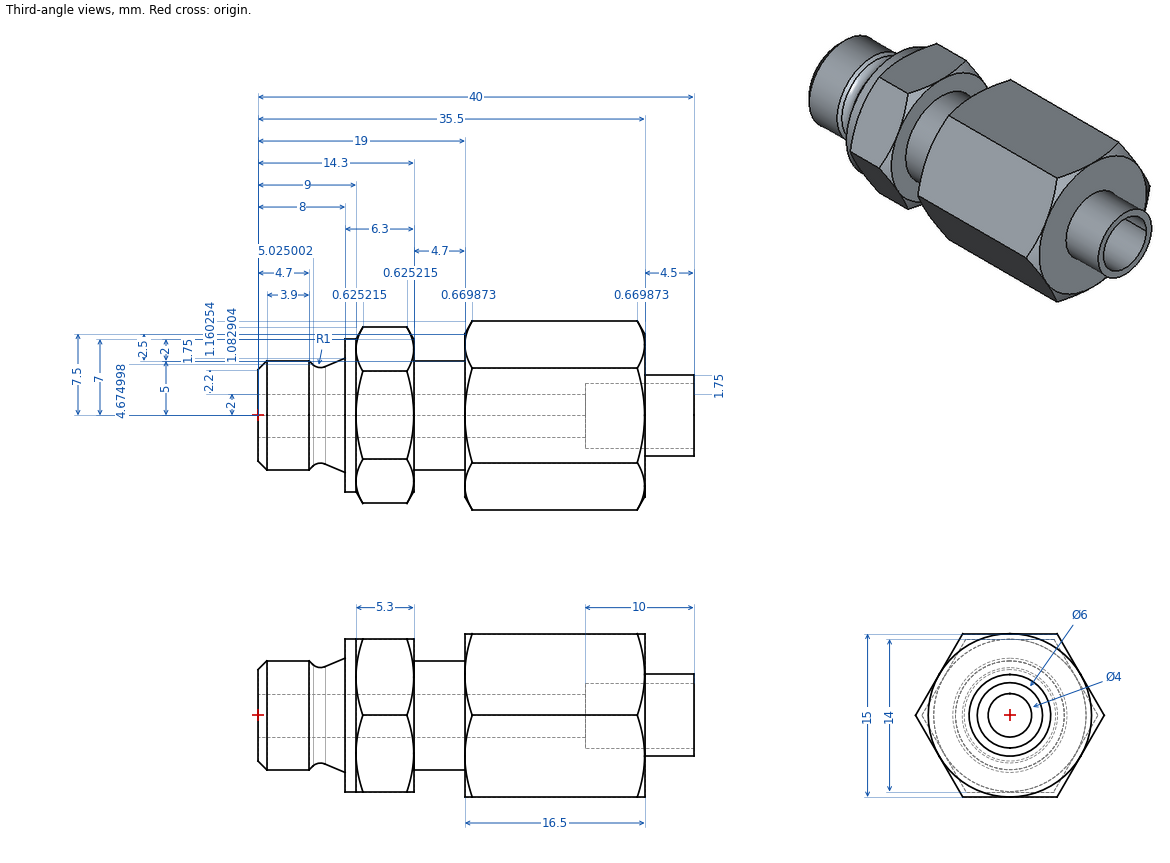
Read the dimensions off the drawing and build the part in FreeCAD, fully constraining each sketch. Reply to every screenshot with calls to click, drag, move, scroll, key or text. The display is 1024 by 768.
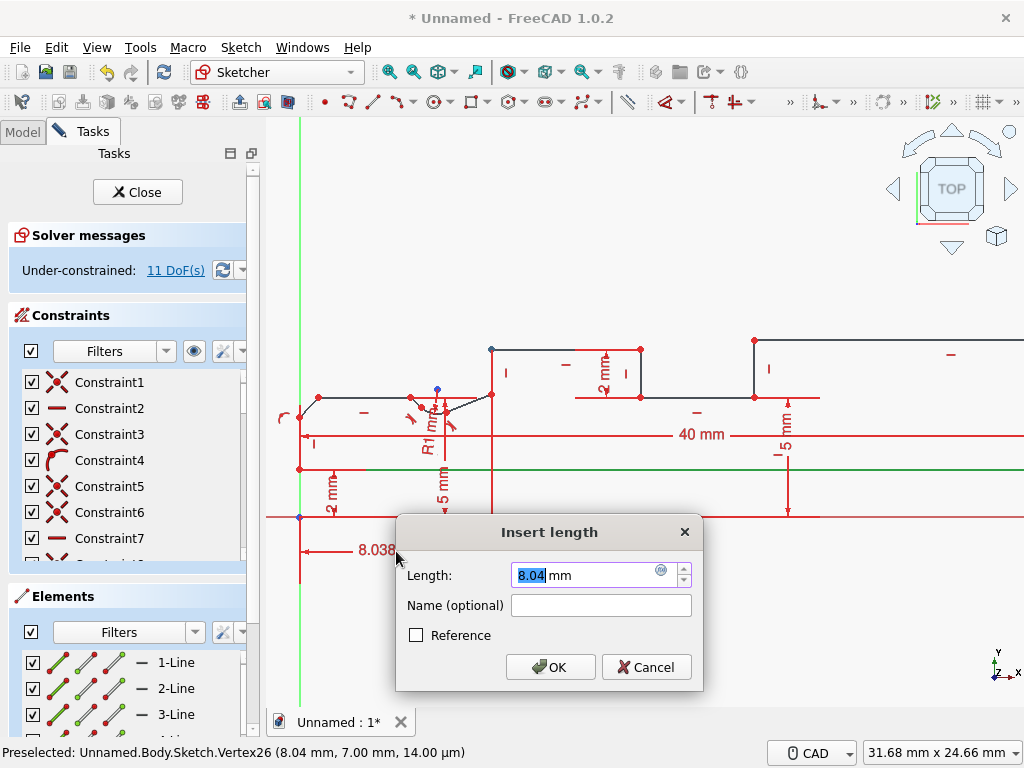
text(8)
key(Return)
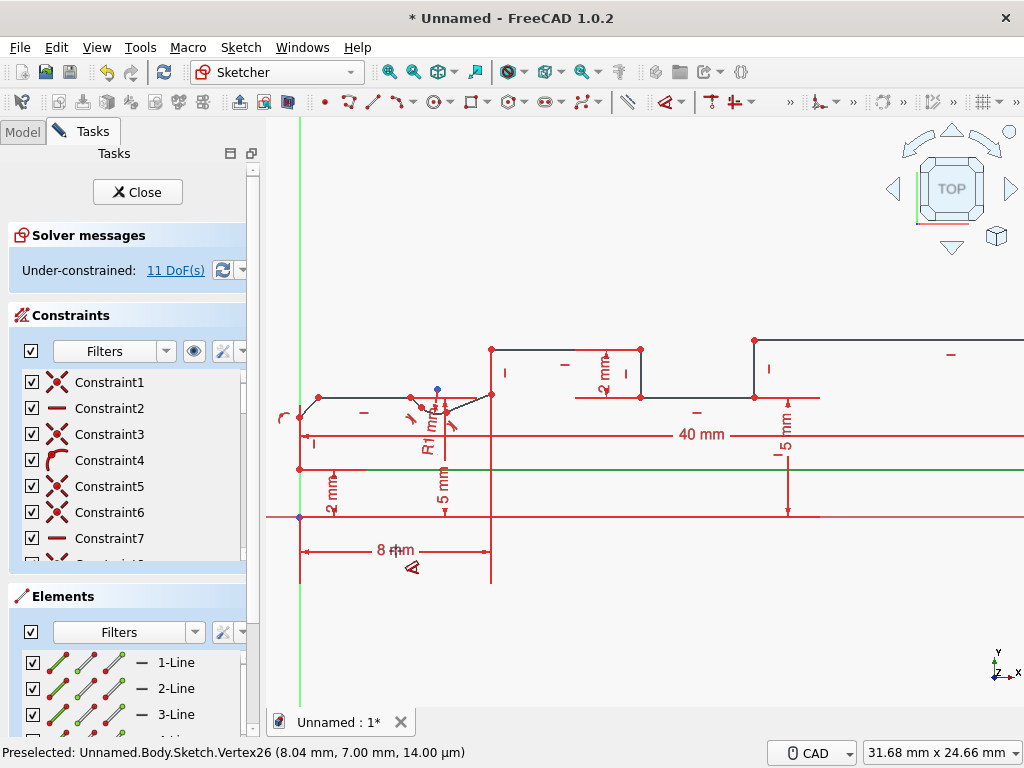
click(383, 398)
click(365, 364)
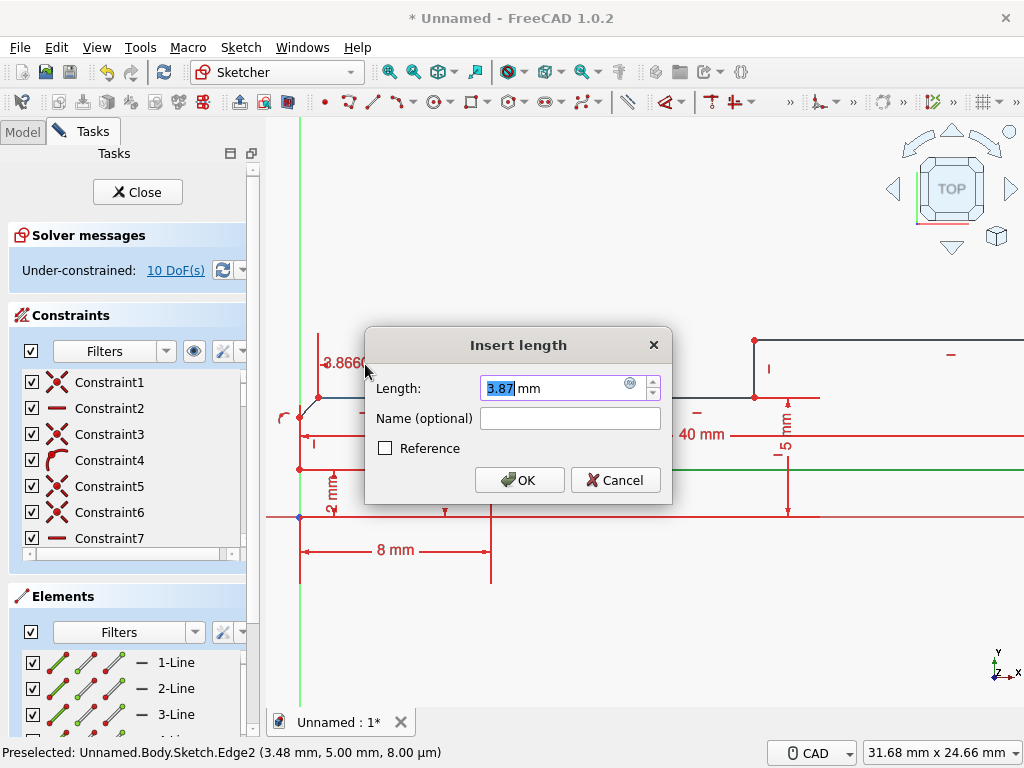
text(3.9)
key(Return)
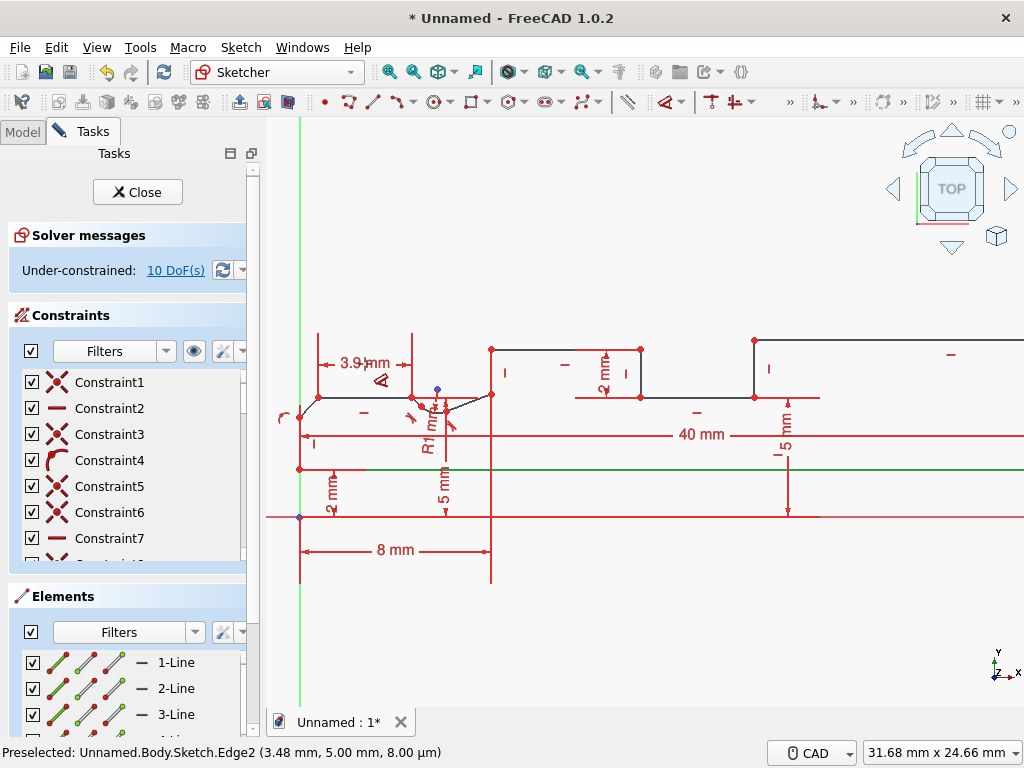
click(300, 433)
click(334, 444)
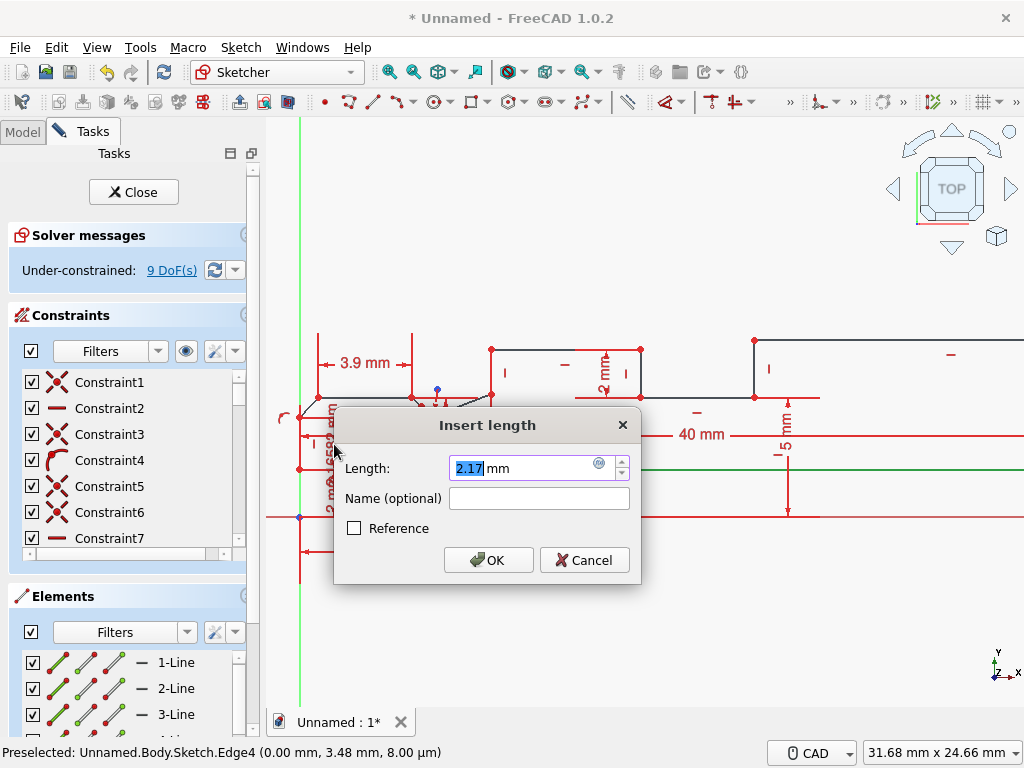
text(2.2)
key(Return)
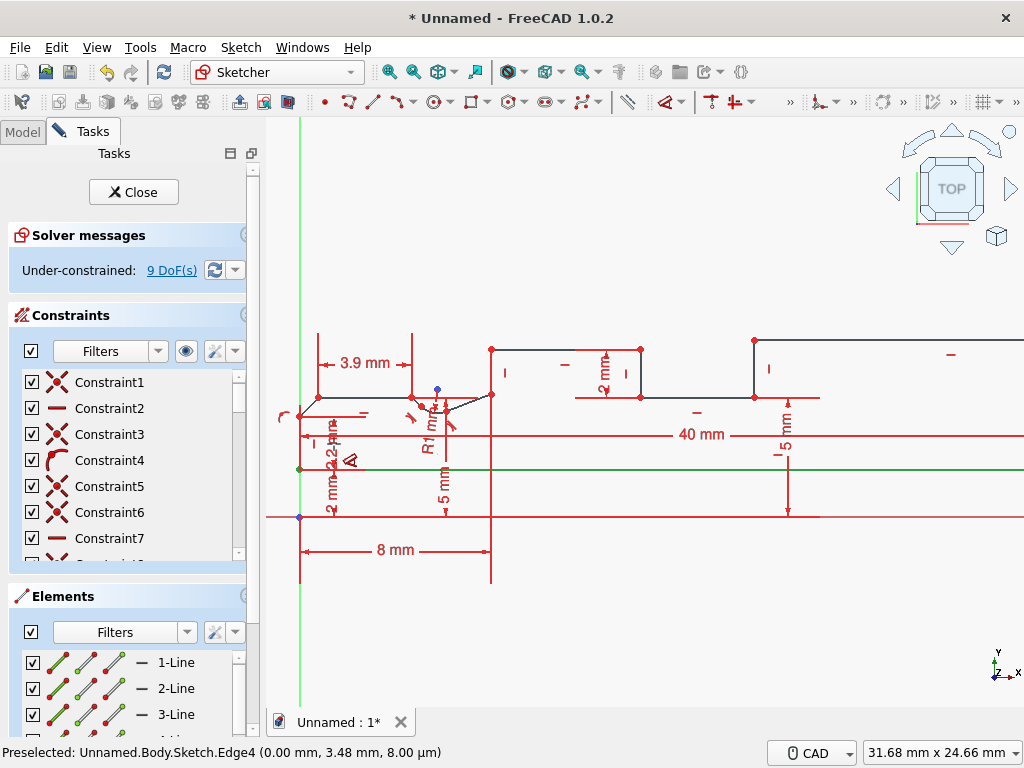
scroll(412, 399, down, 4)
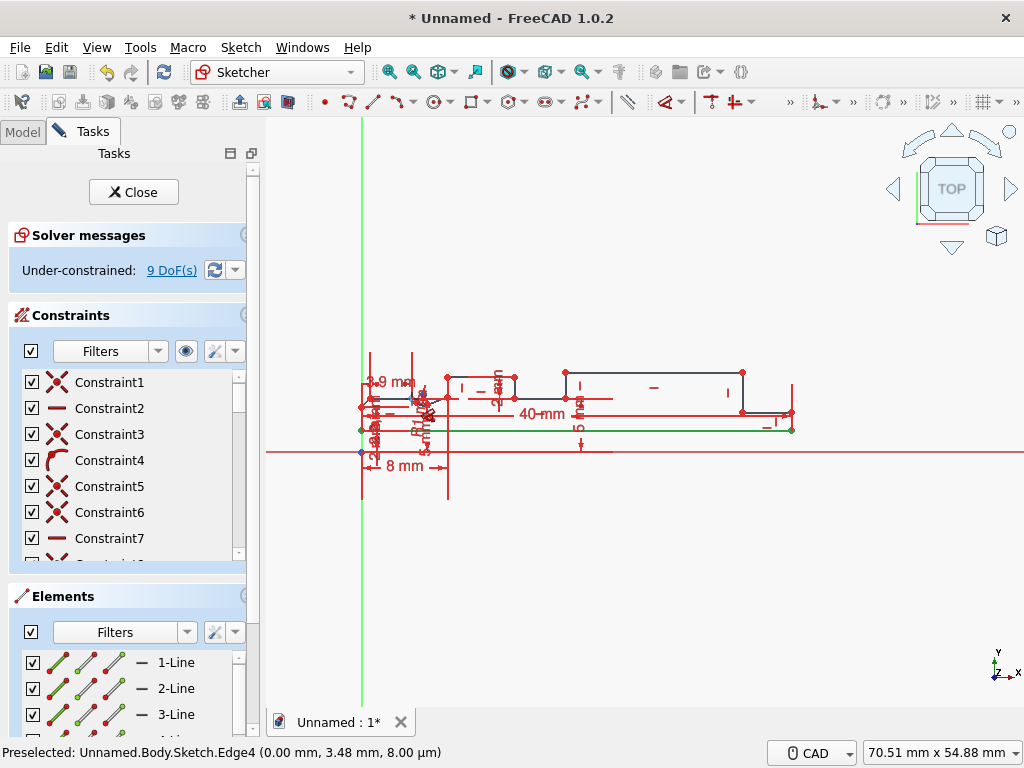
click(777, 413)
click(767, 379)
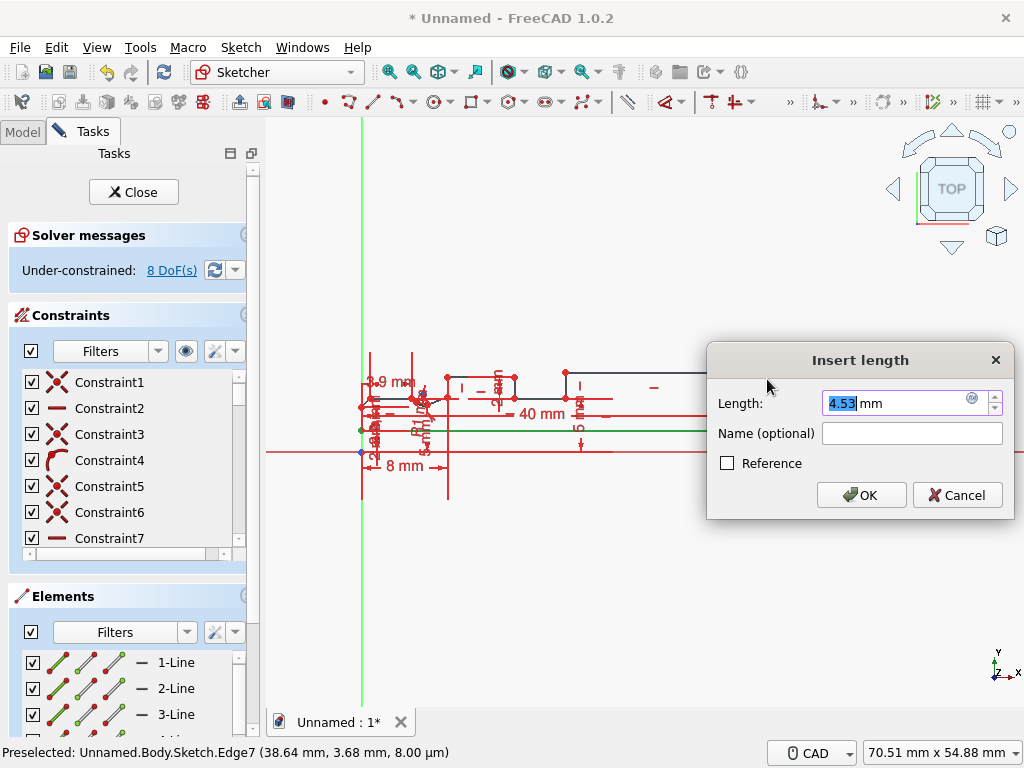
text(4.5)
key(Return)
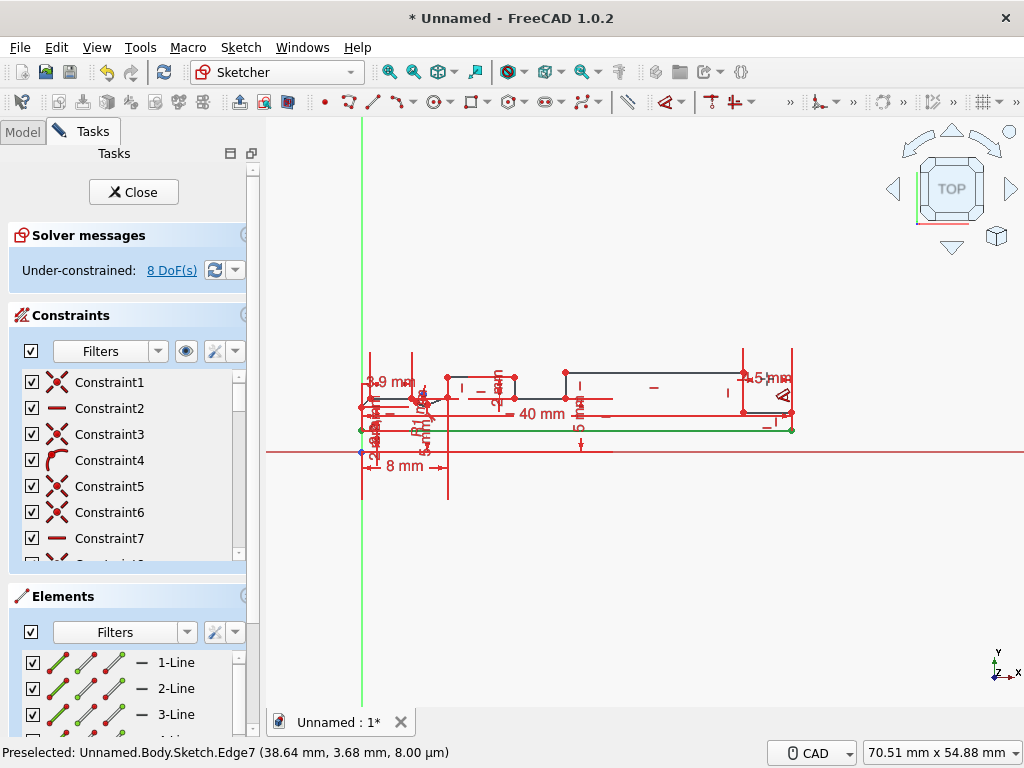
scroll(566, 383, up, 2)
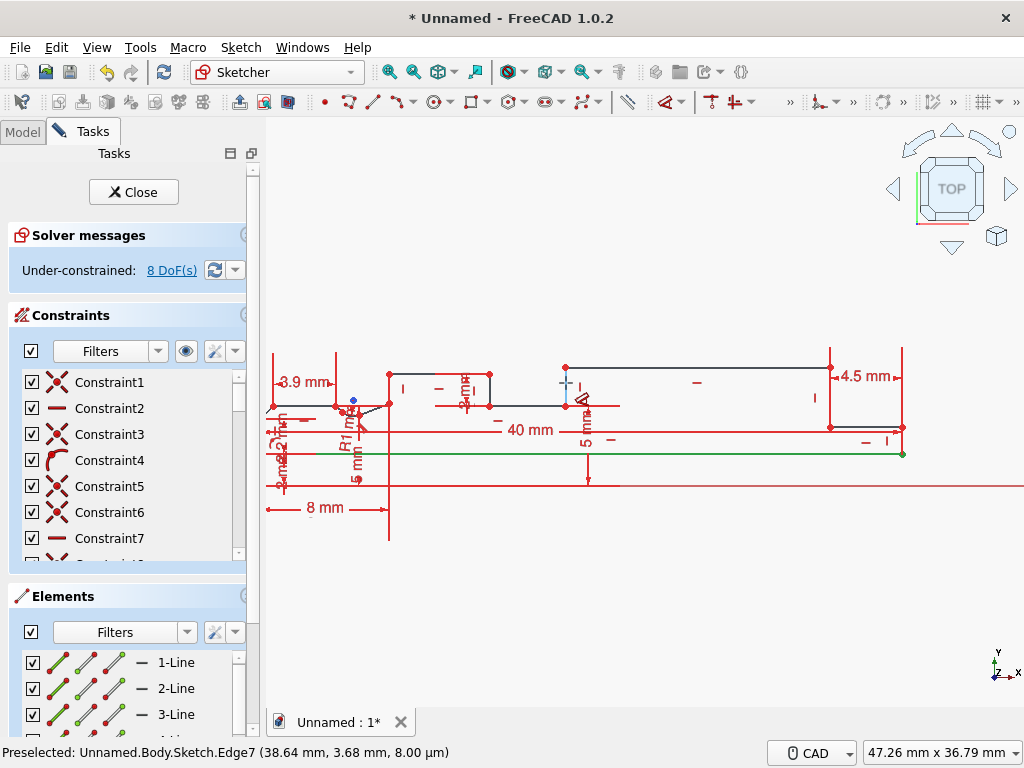
click(566, 383)
click(600, 387)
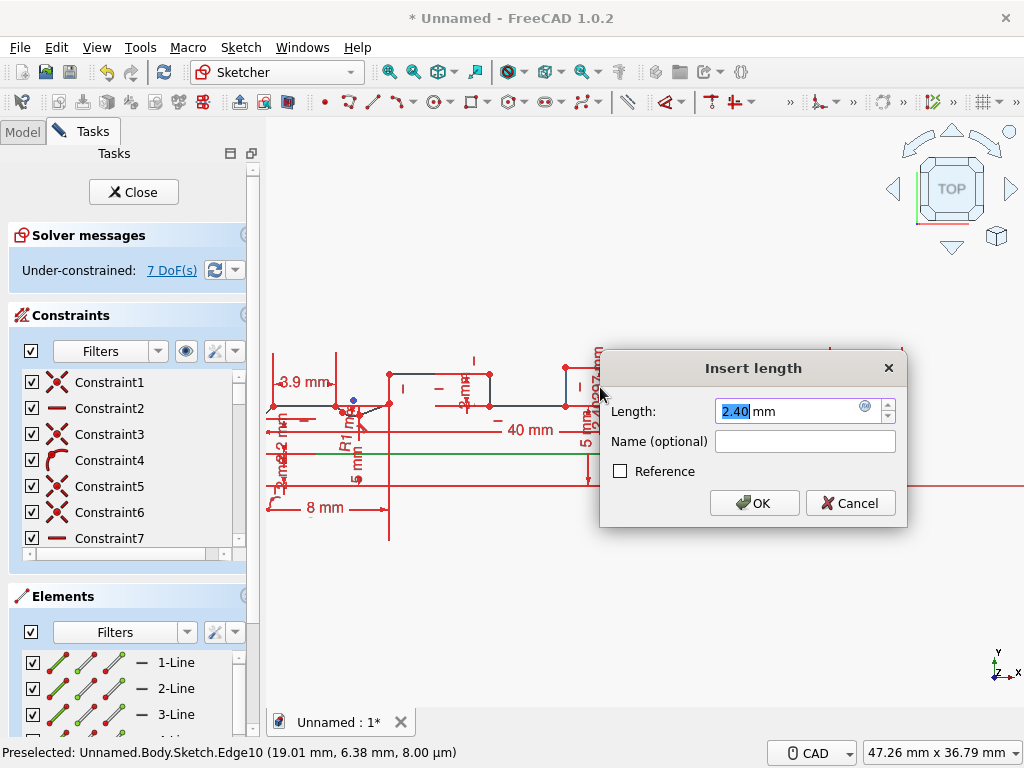
text(2.5)
key(Return)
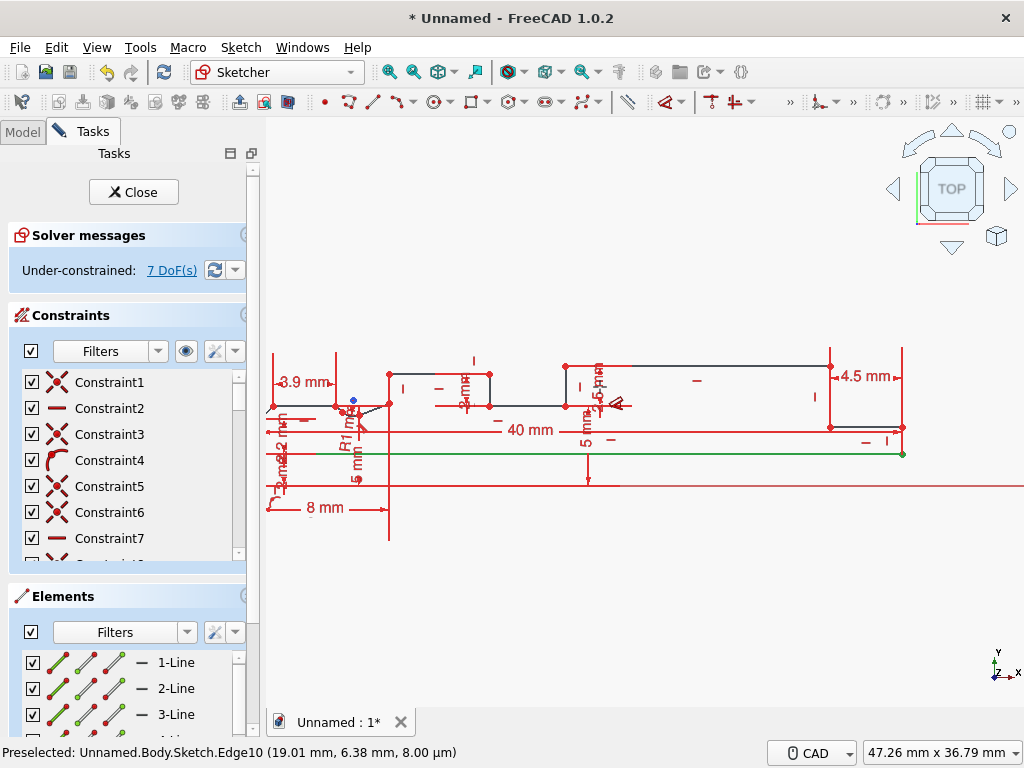
click(543, 406)
click(528, 348)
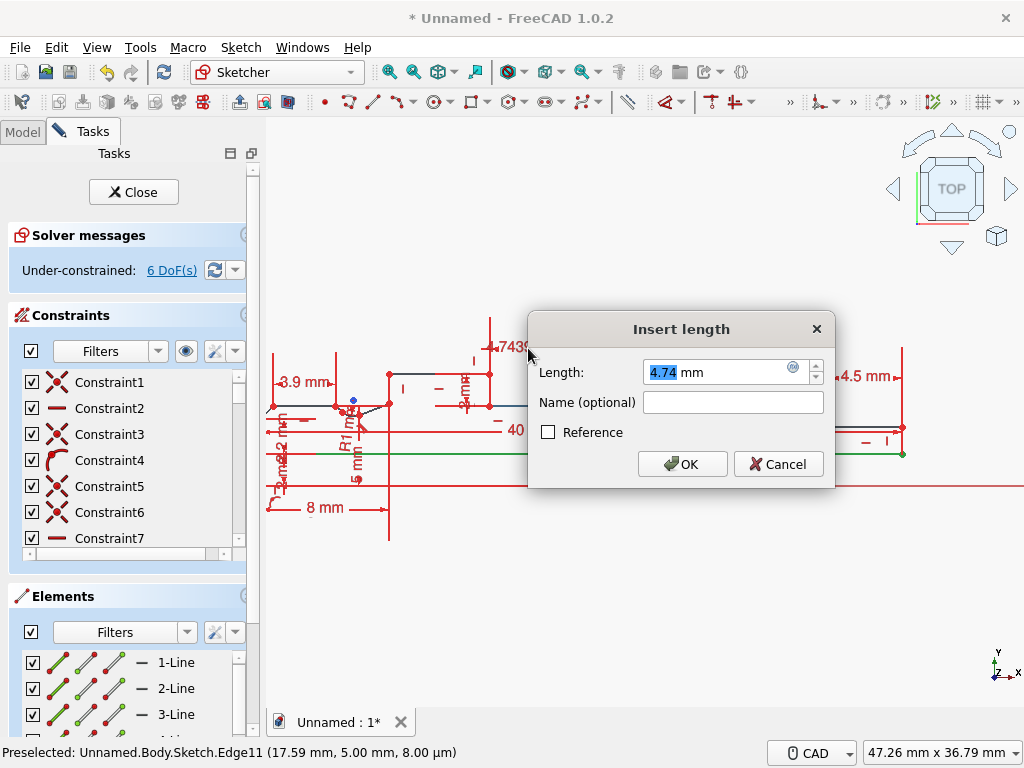
text(4.7)
key(Return)